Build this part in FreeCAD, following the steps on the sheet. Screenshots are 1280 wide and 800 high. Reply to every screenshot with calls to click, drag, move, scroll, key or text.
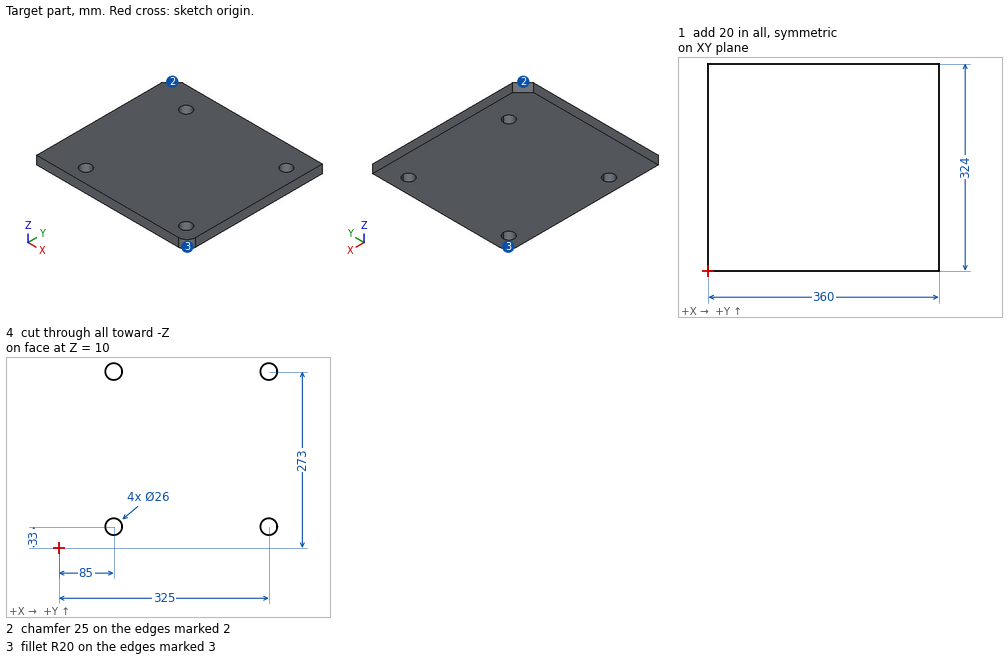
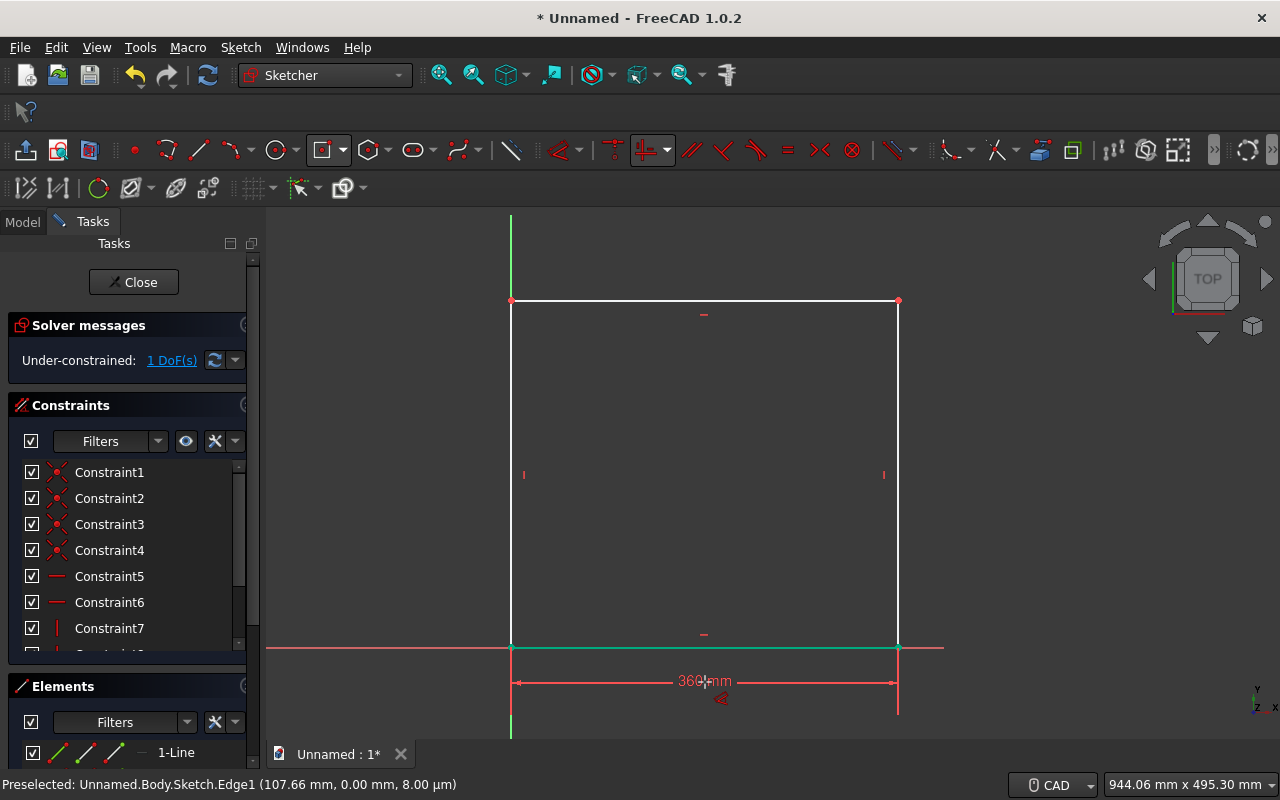
click(898, 544)
click(932, 474)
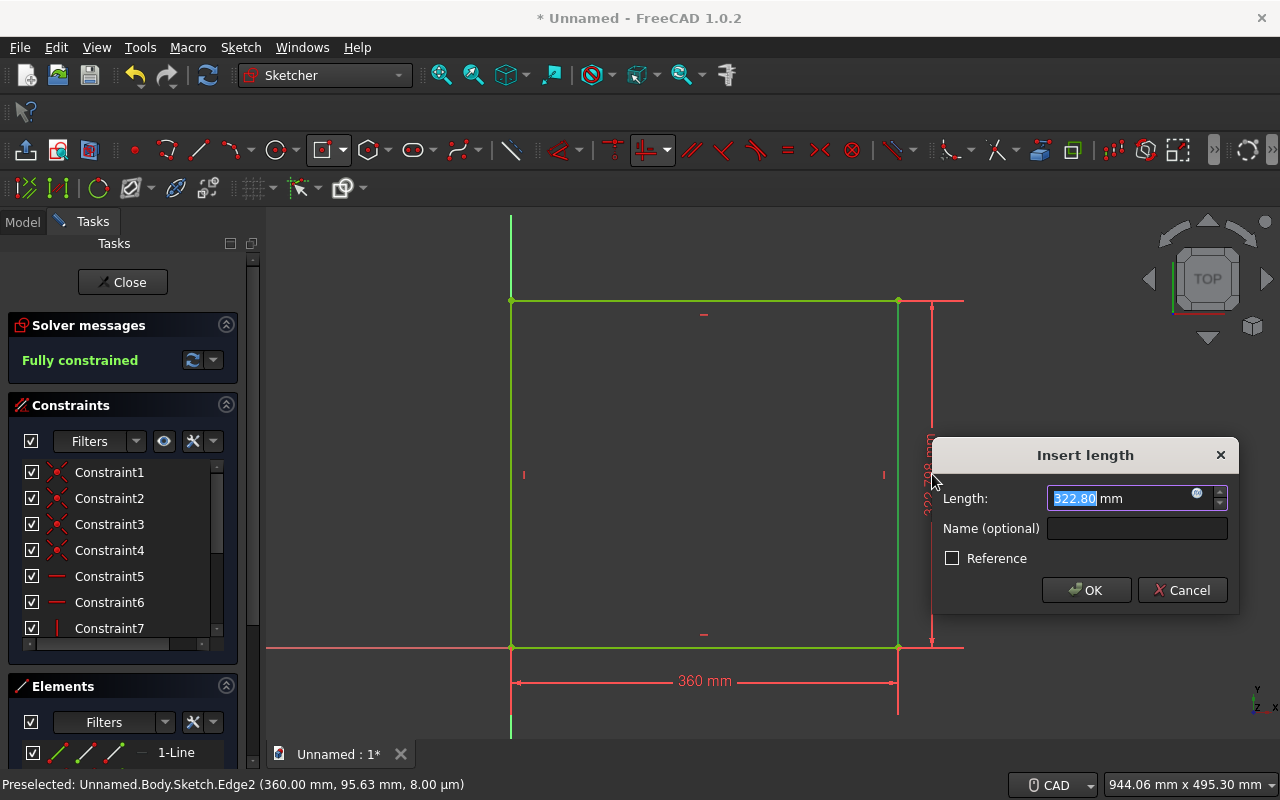
text(324)
key(Return)
key(Escape)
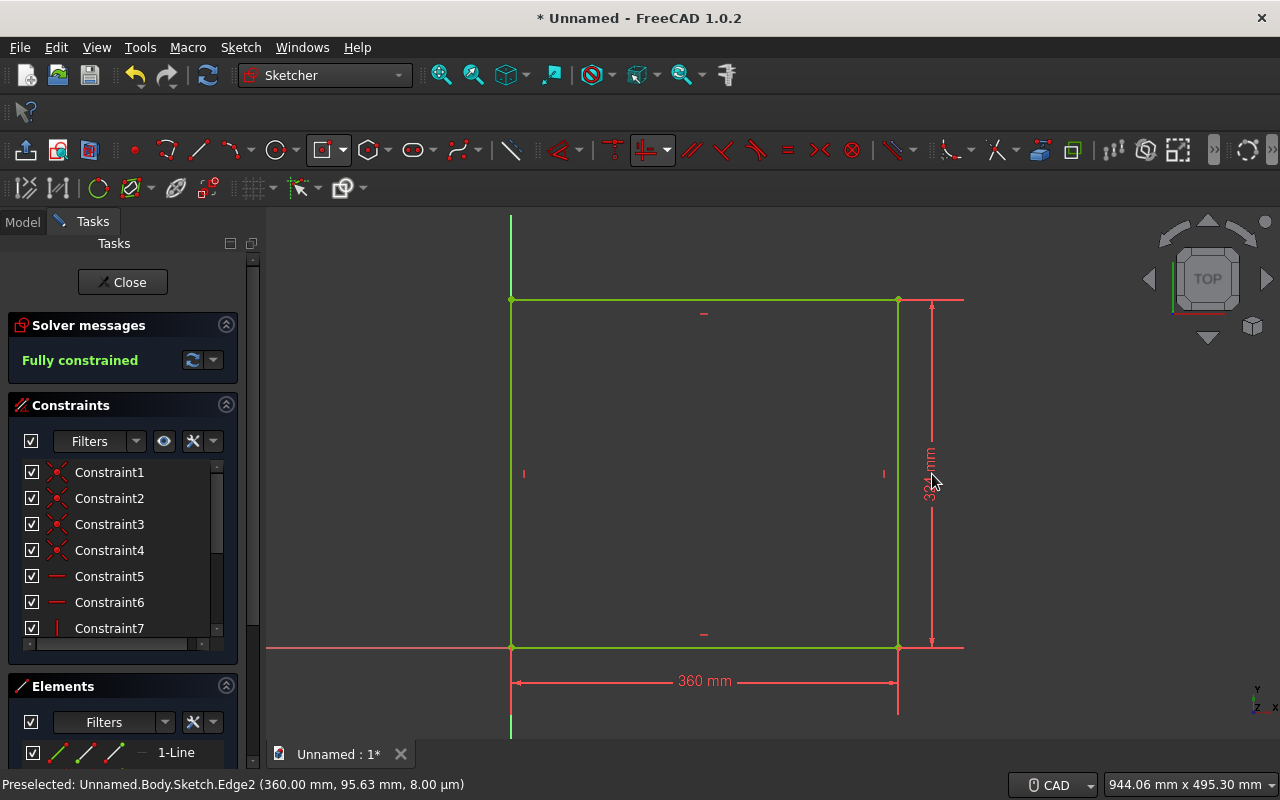
click(123, 282)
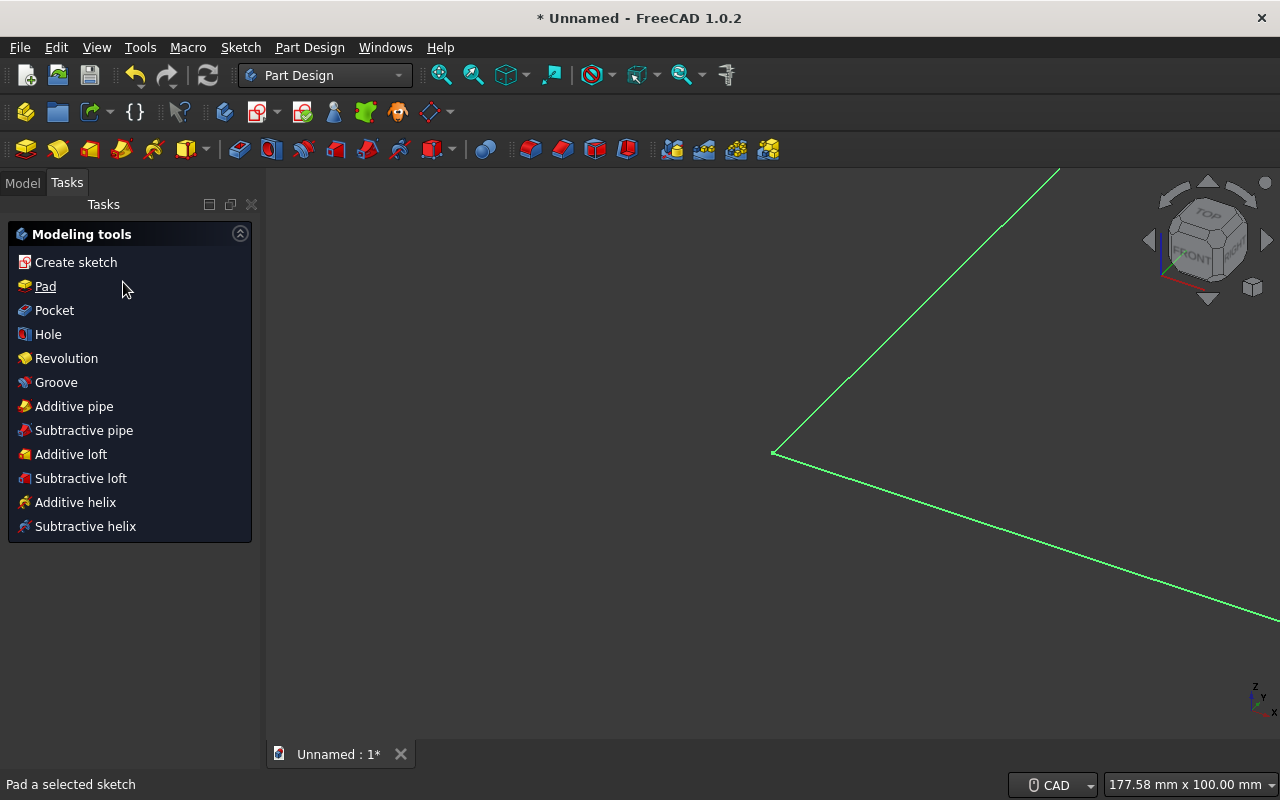
click(26, 150)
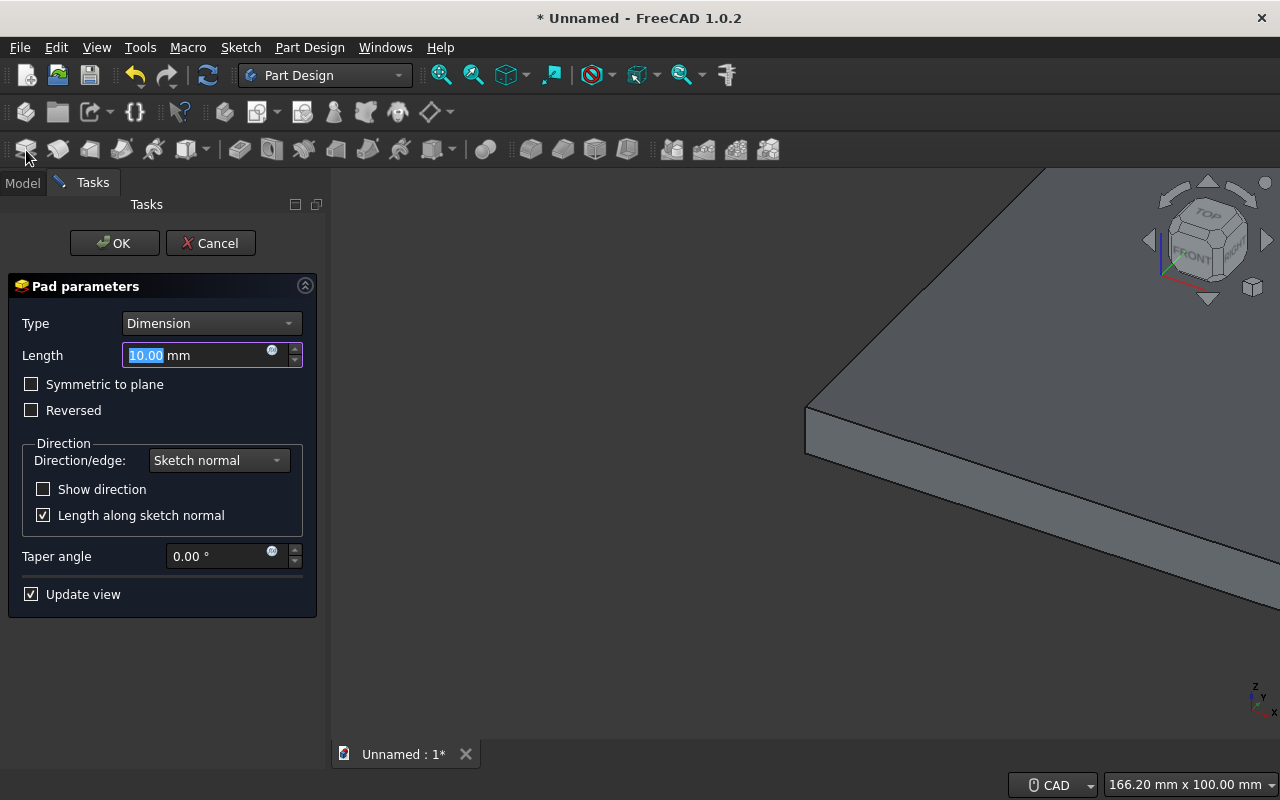
text(20)
key(Tab)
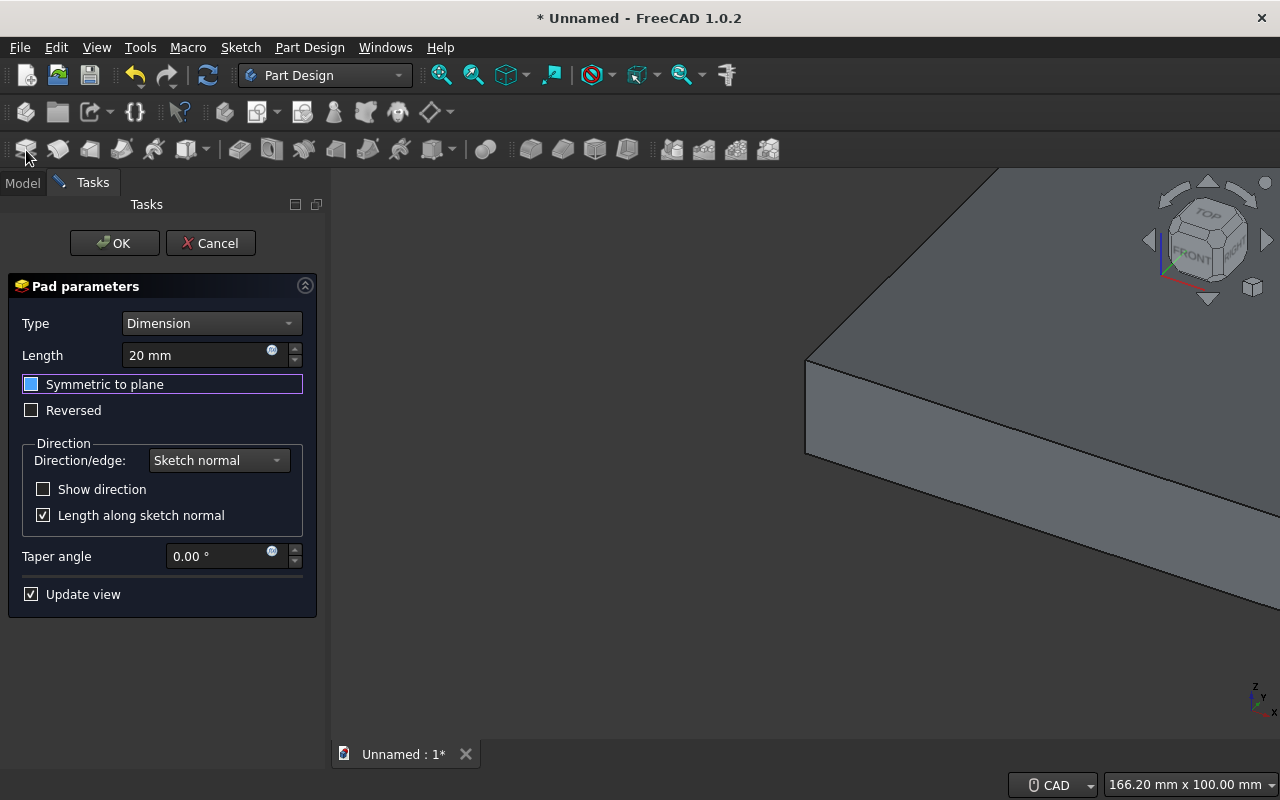
click(30, 384)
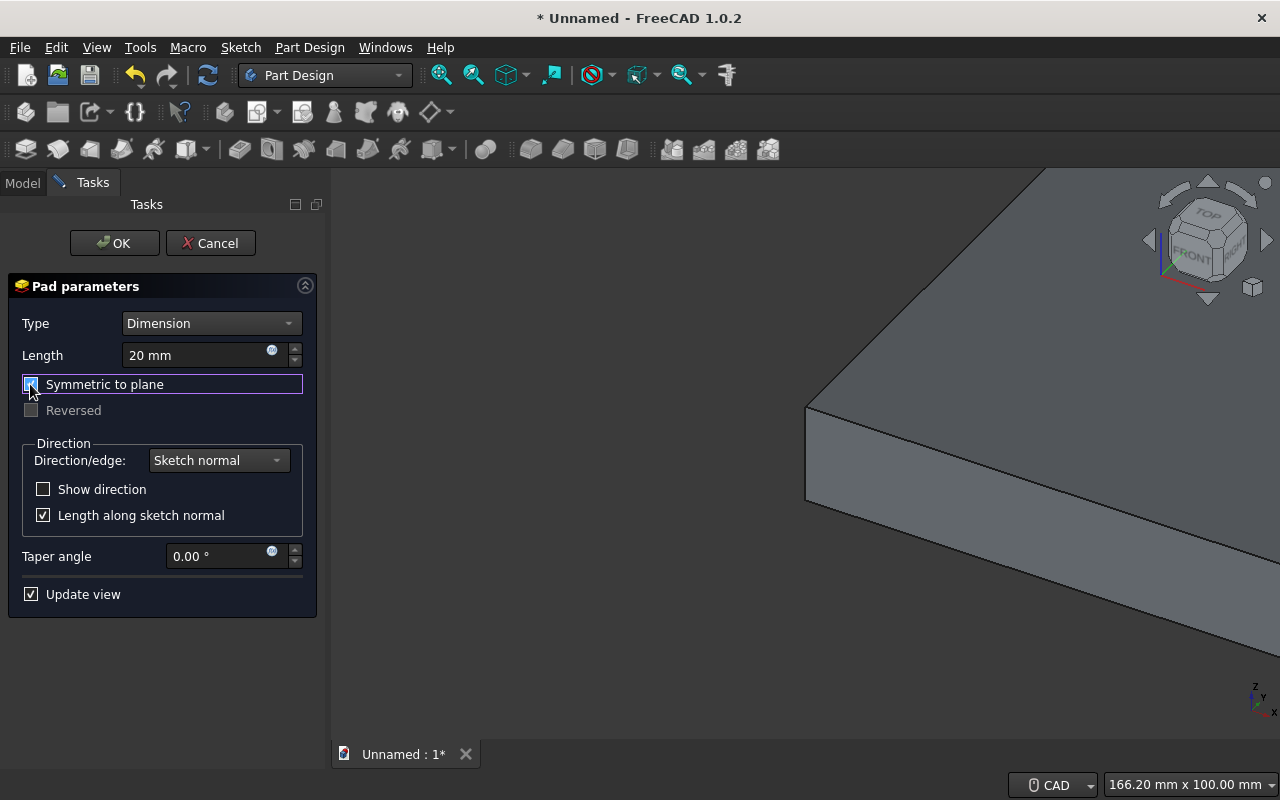
click(115, 243)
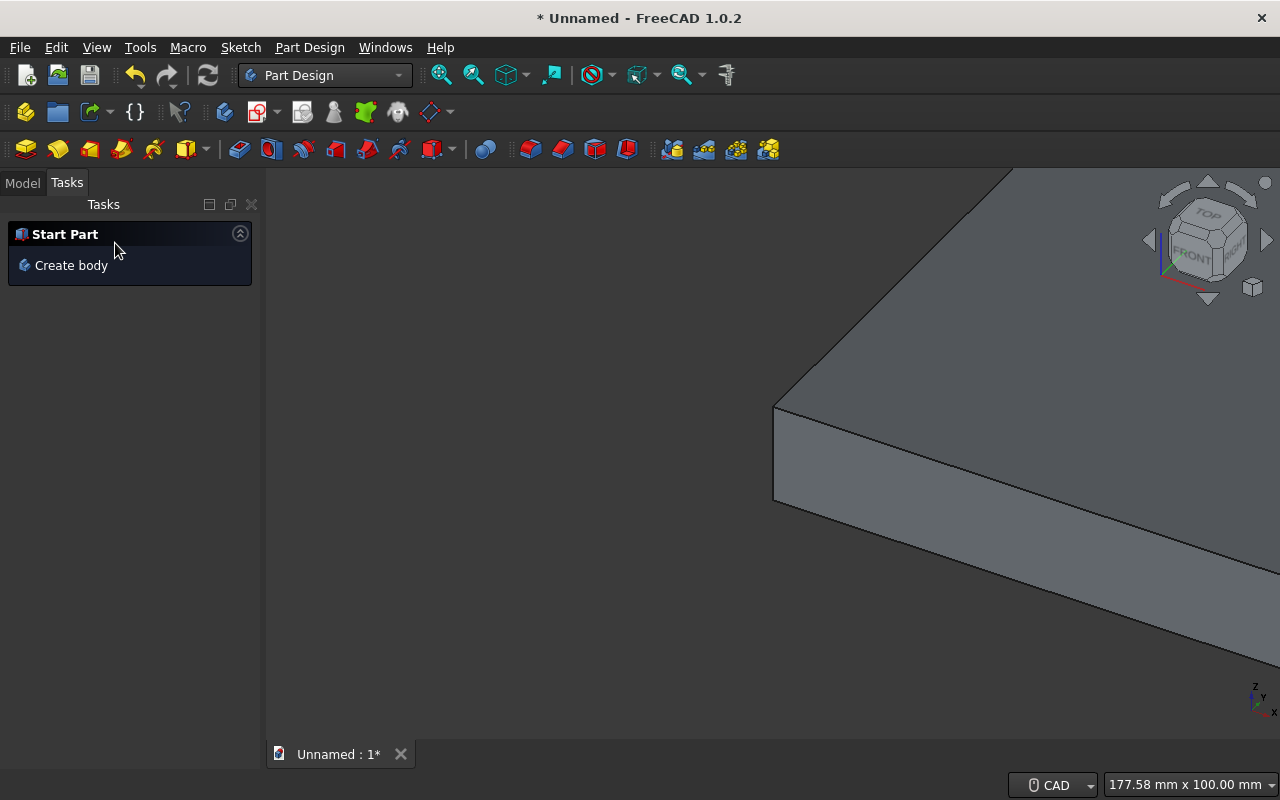
click(442, 76)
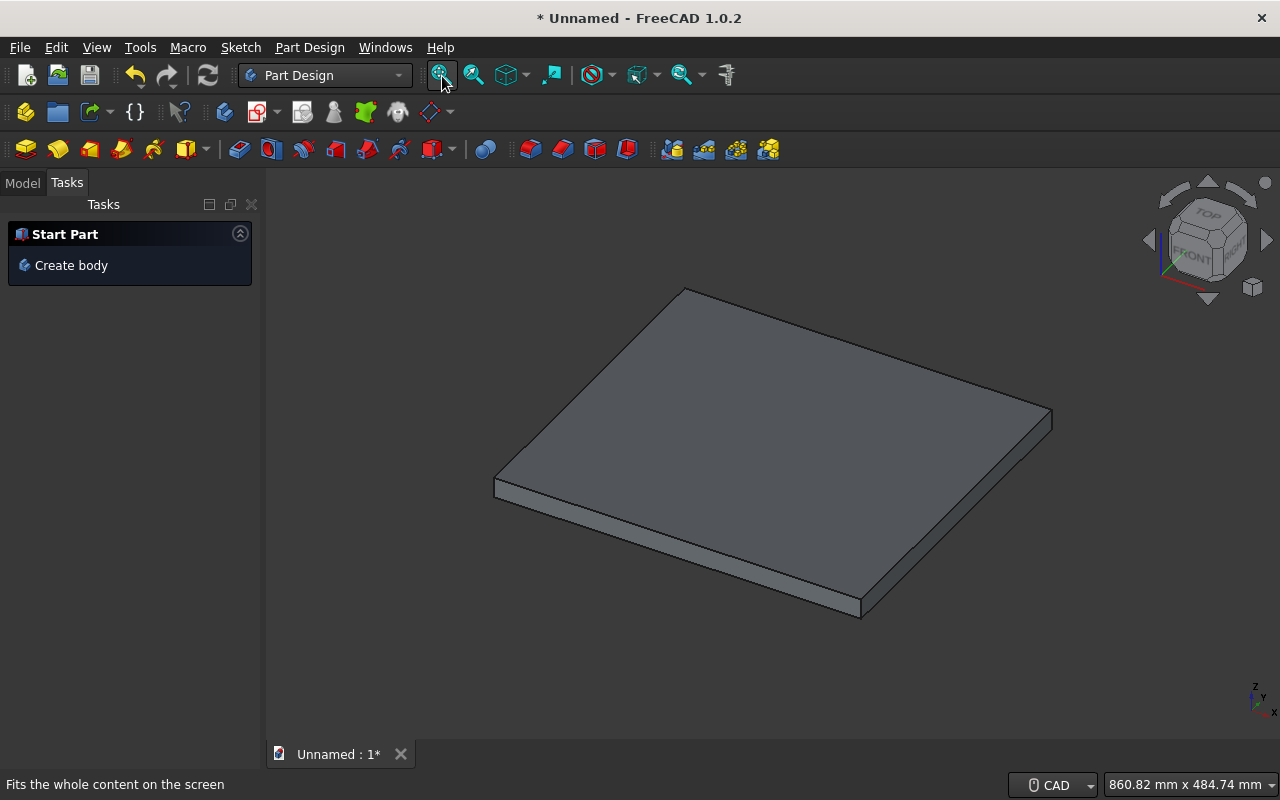
key(0)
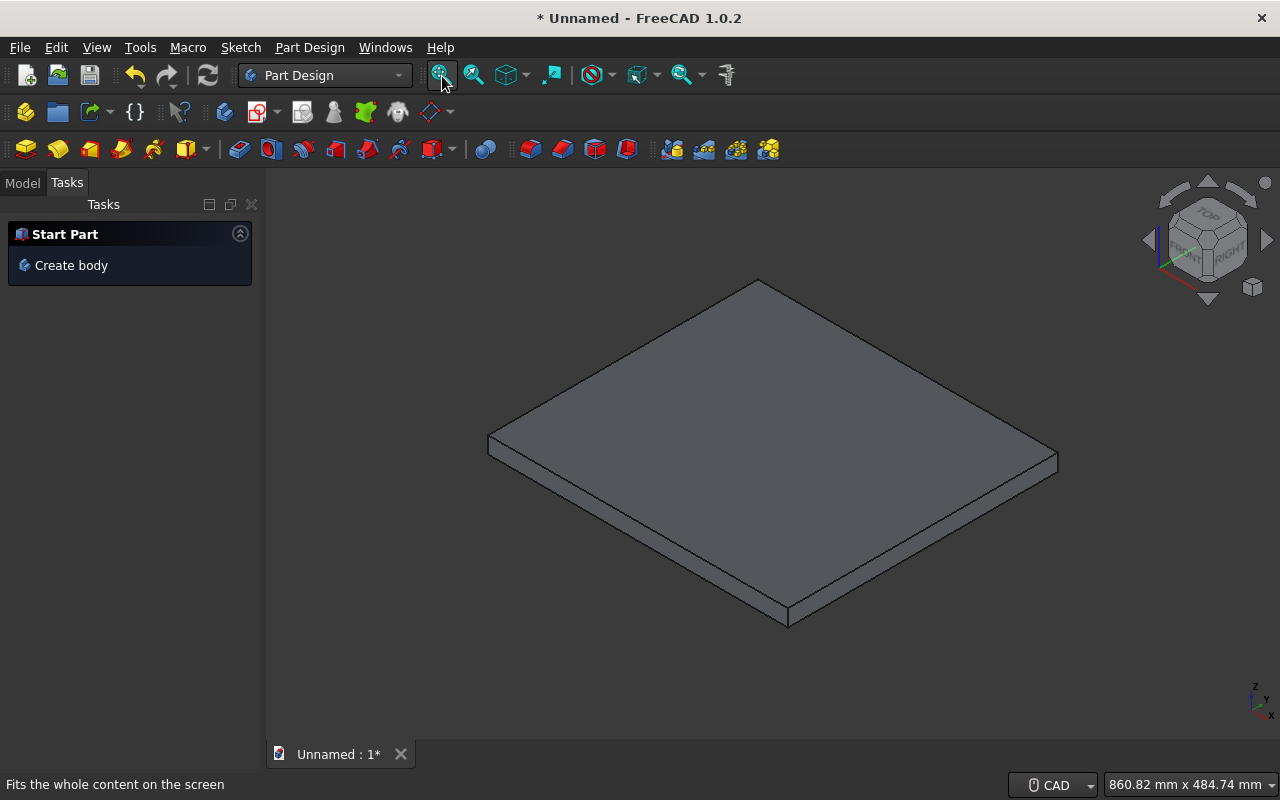
key(2)